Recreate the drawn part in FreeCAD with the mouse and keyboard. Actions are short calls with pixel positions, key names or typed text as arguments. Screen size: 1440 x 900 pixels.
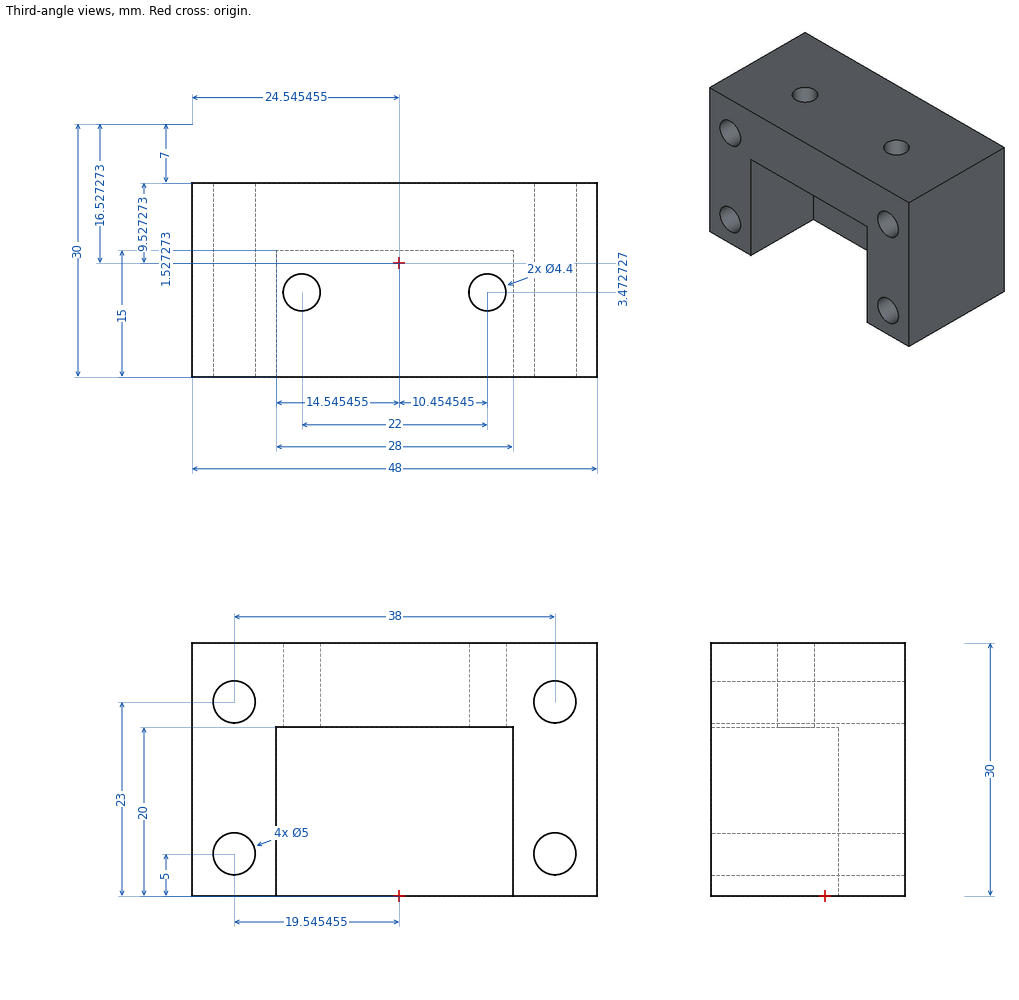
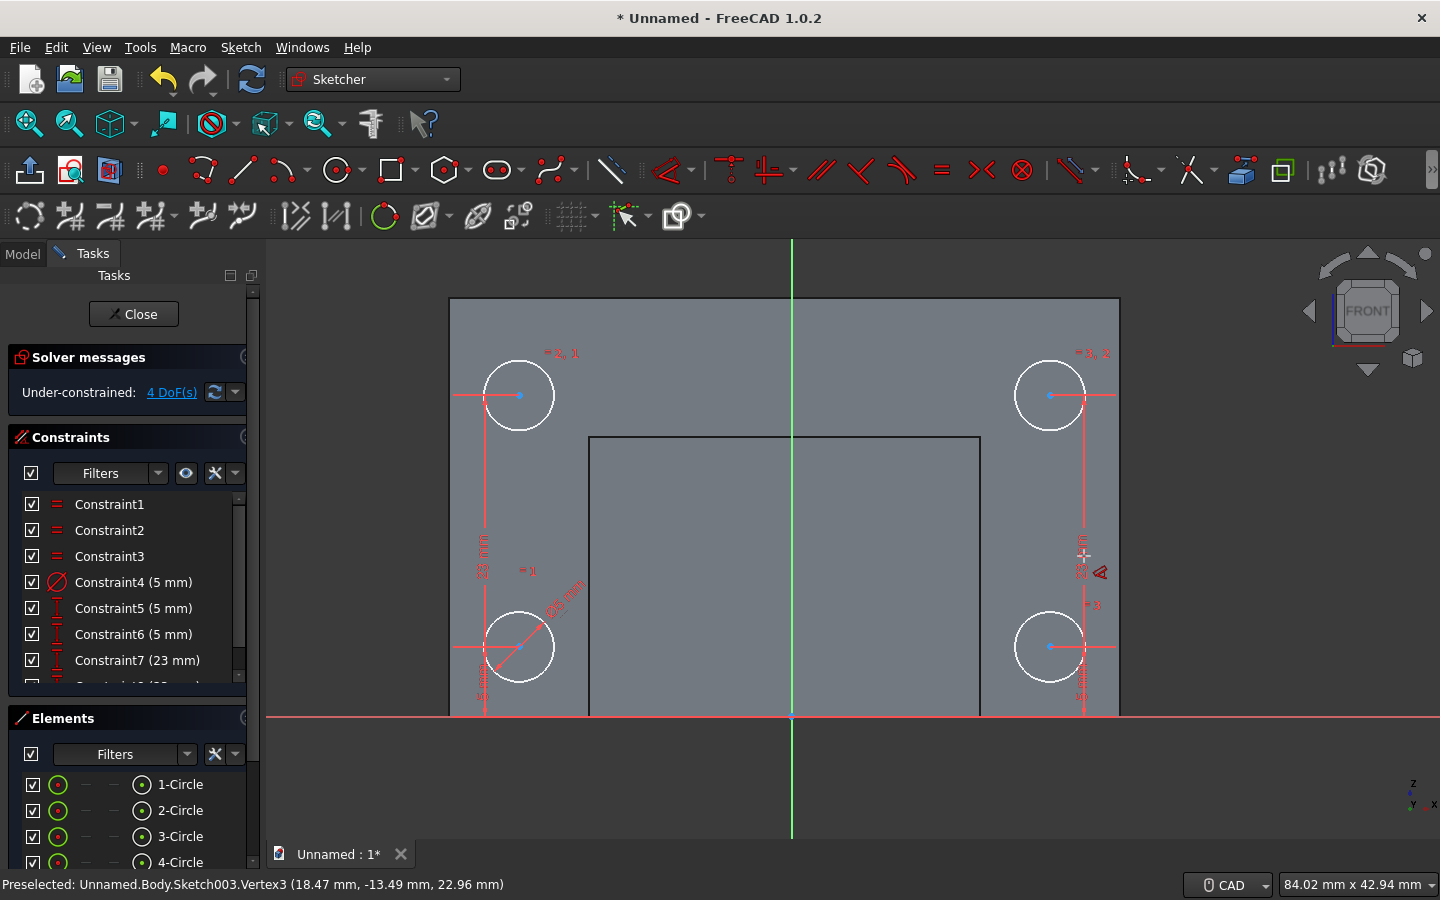
click(519, 395)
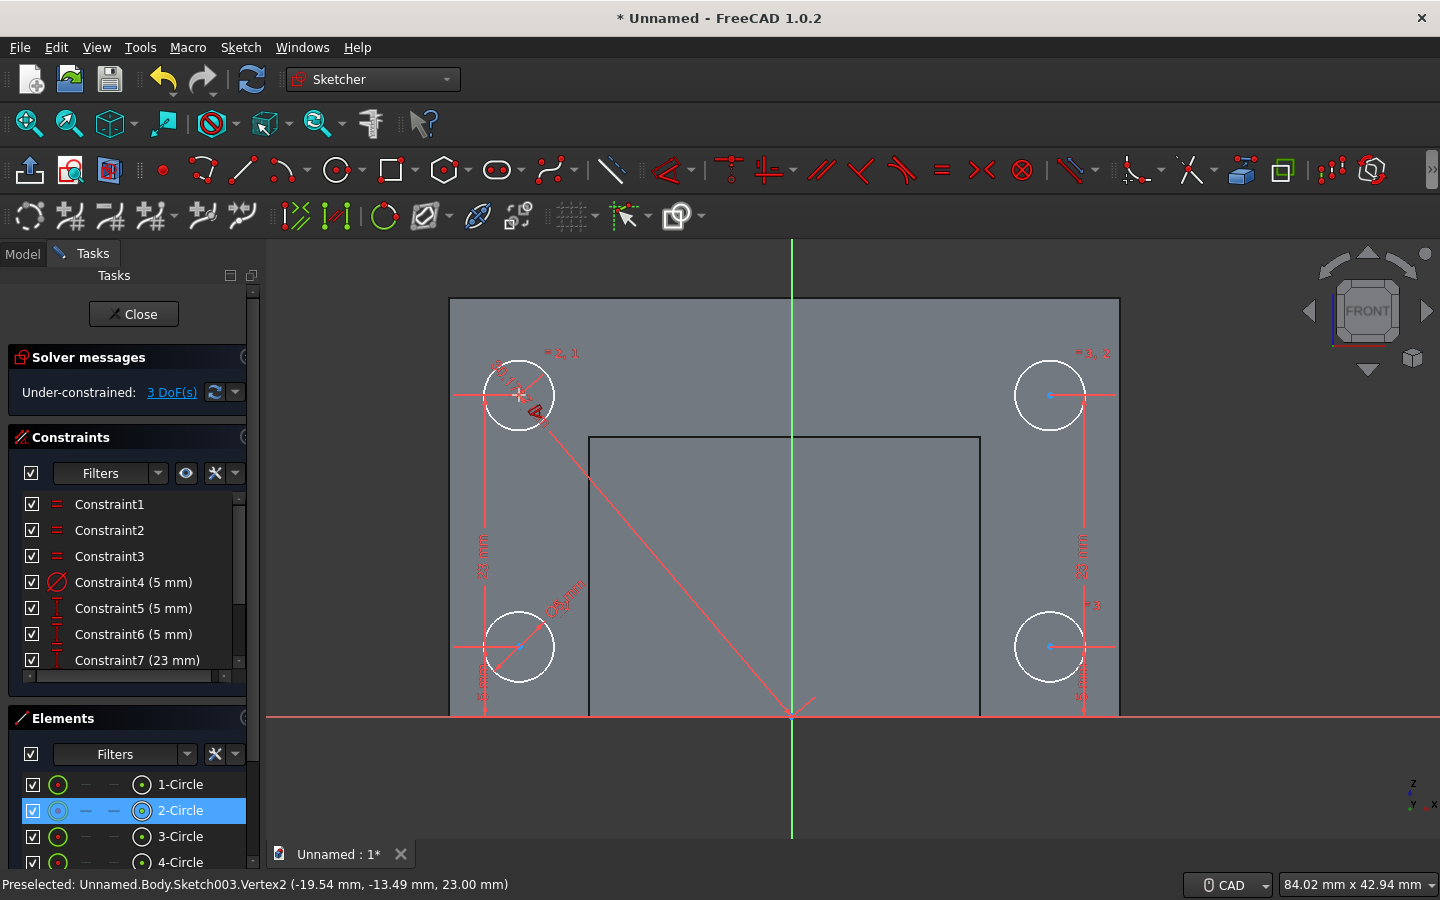
click(1050, 395)
click(662, 361)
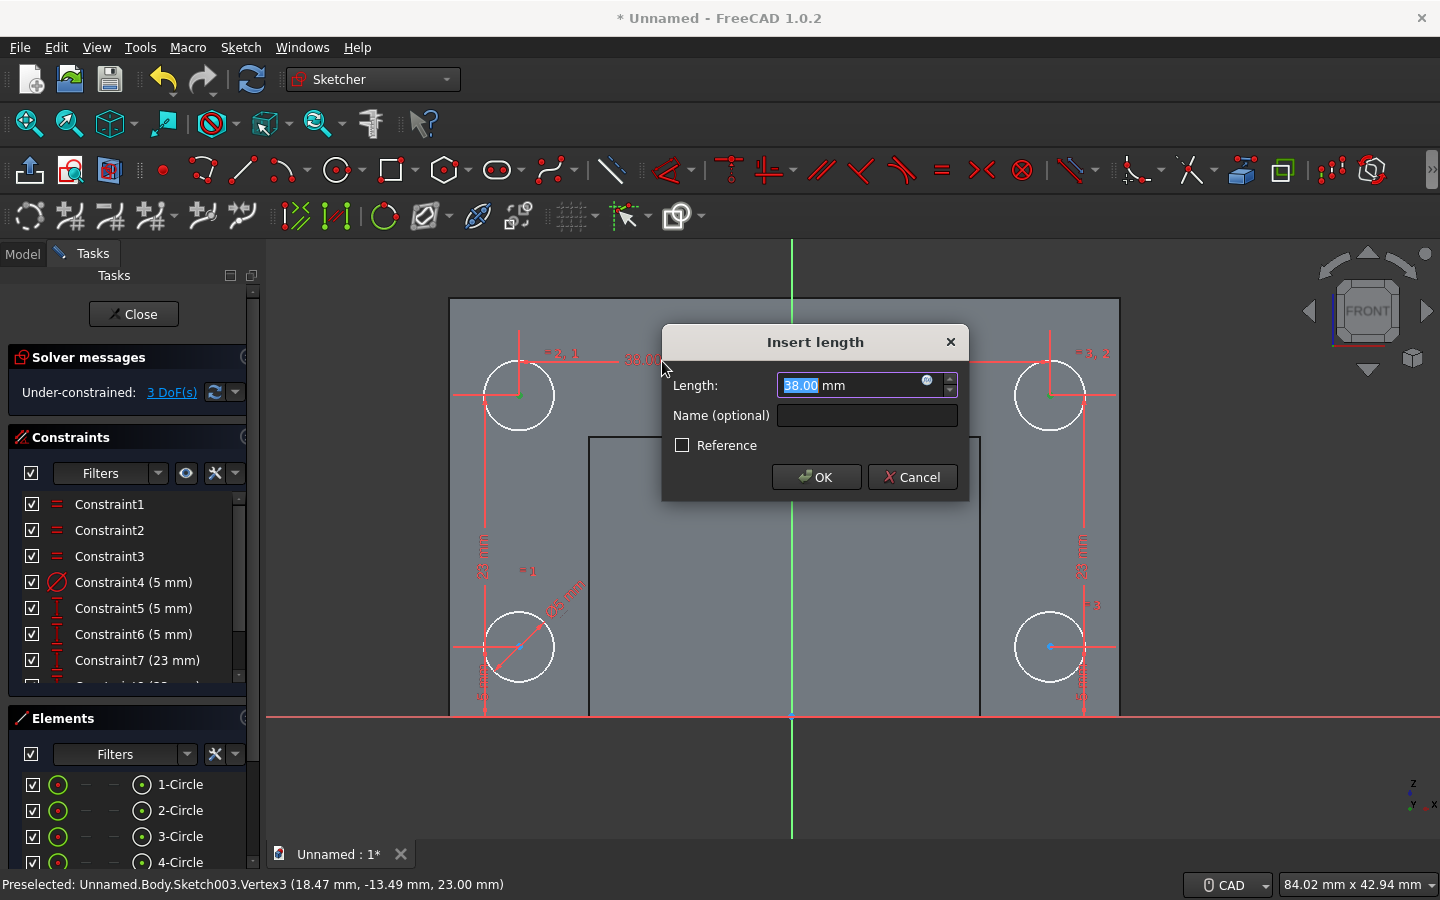
text(38)
key(Return)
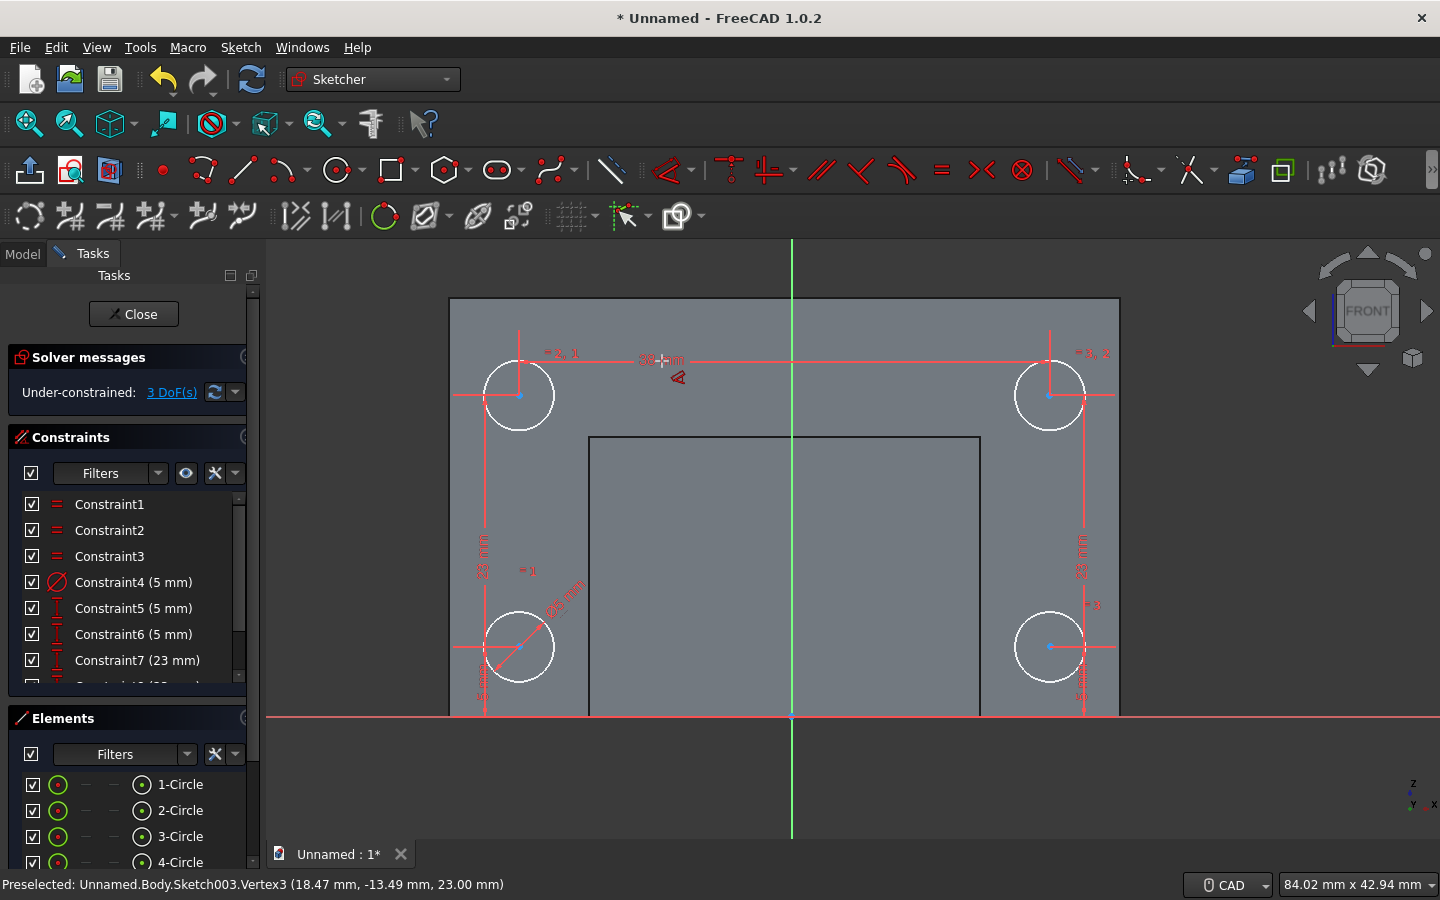
click(519, 647)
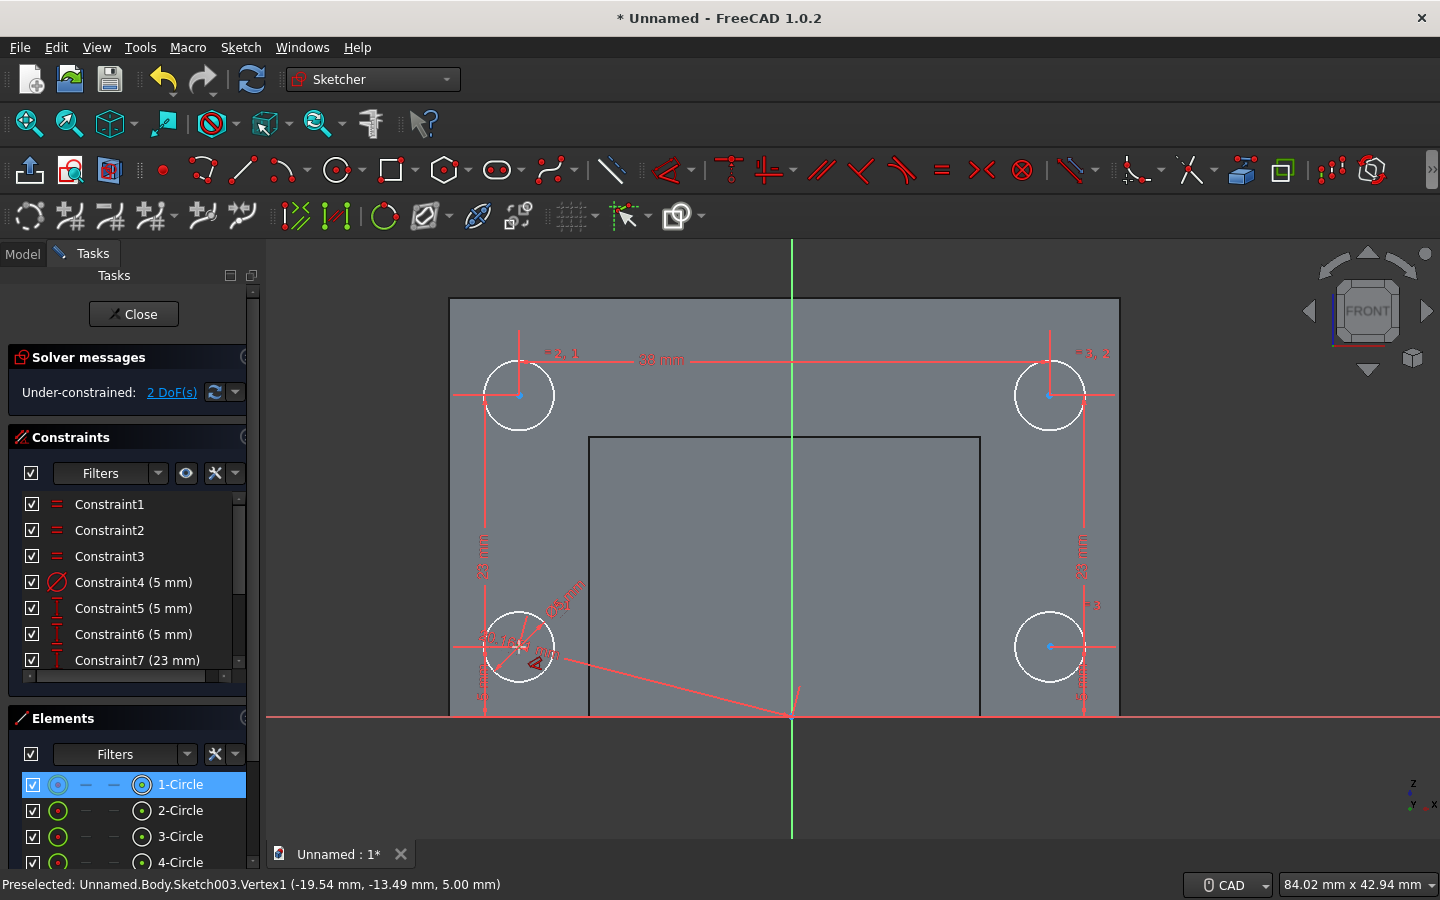
click(1050, 395)
click(907, 361)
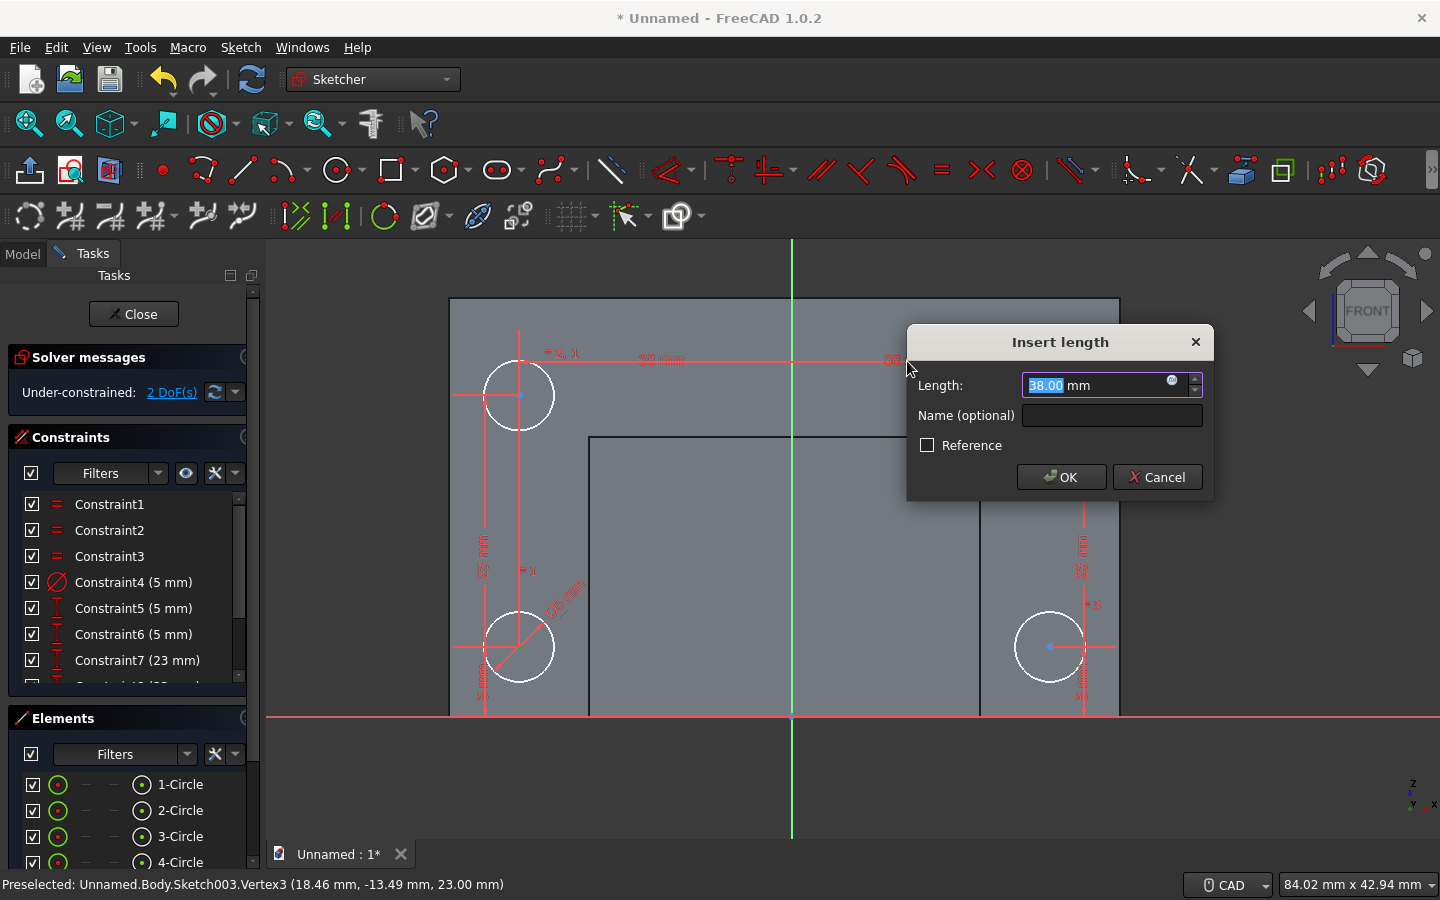
text(38)
key(Return)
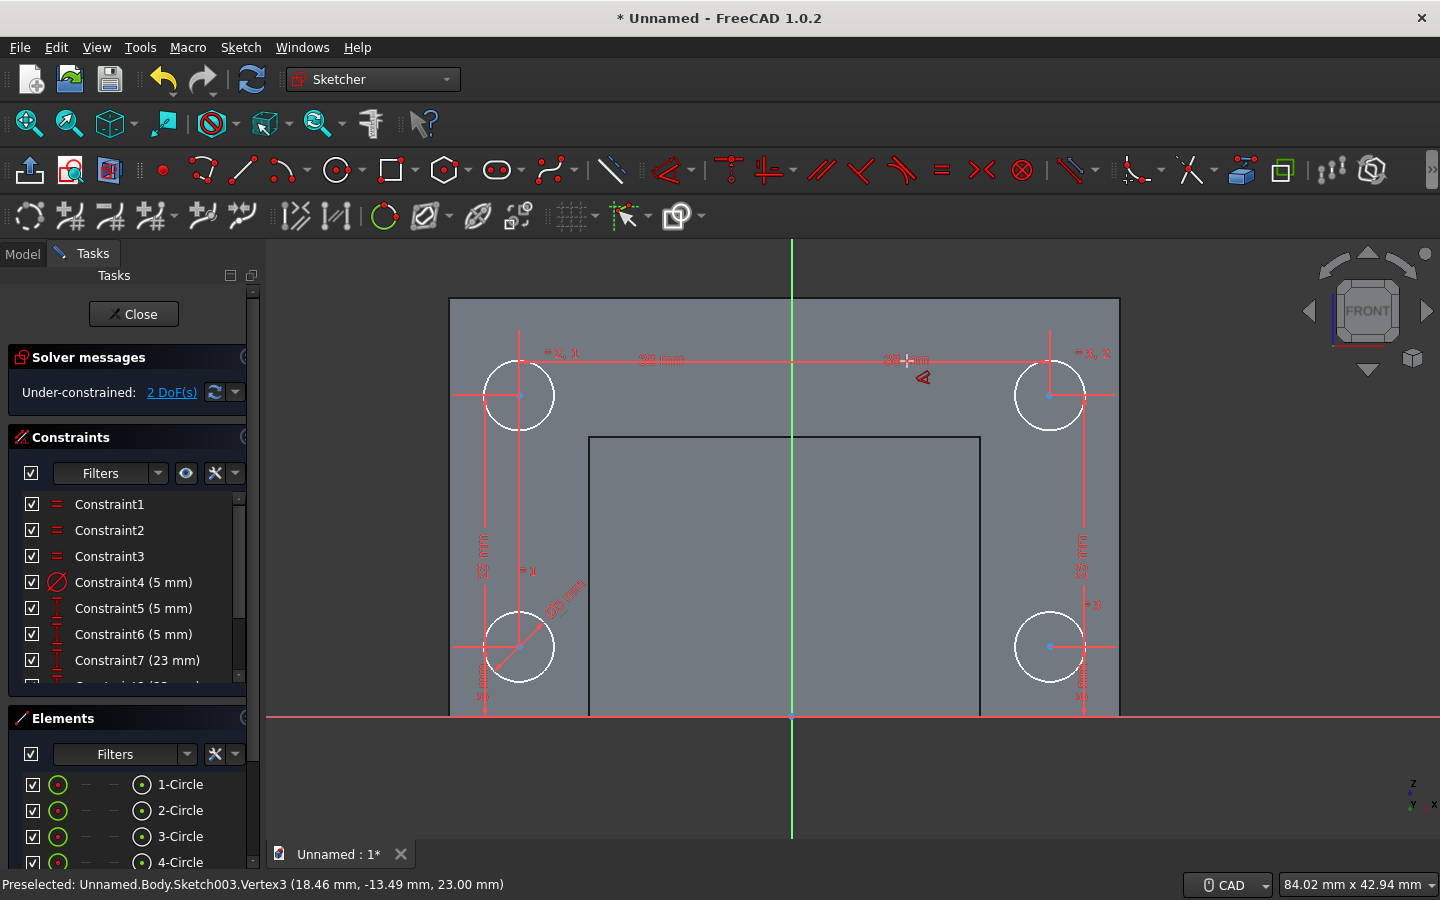
click(519, 647)